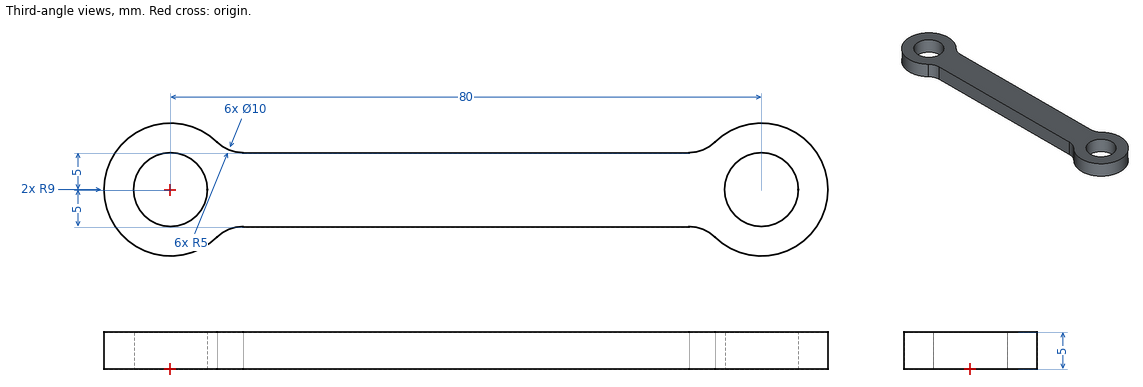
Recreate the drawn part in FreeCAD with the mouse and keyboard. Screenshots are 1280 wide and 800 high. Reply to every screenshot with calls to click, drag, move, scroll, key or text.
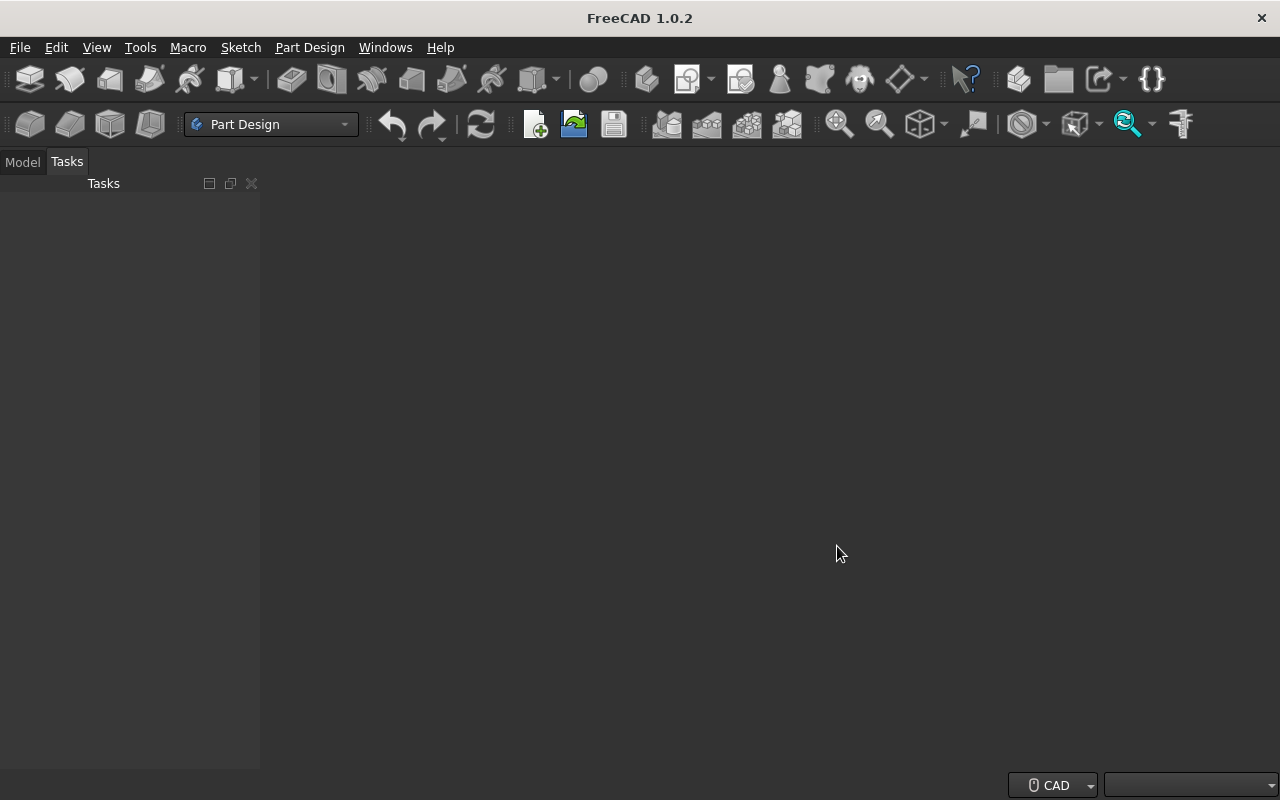
key(ctrl+n)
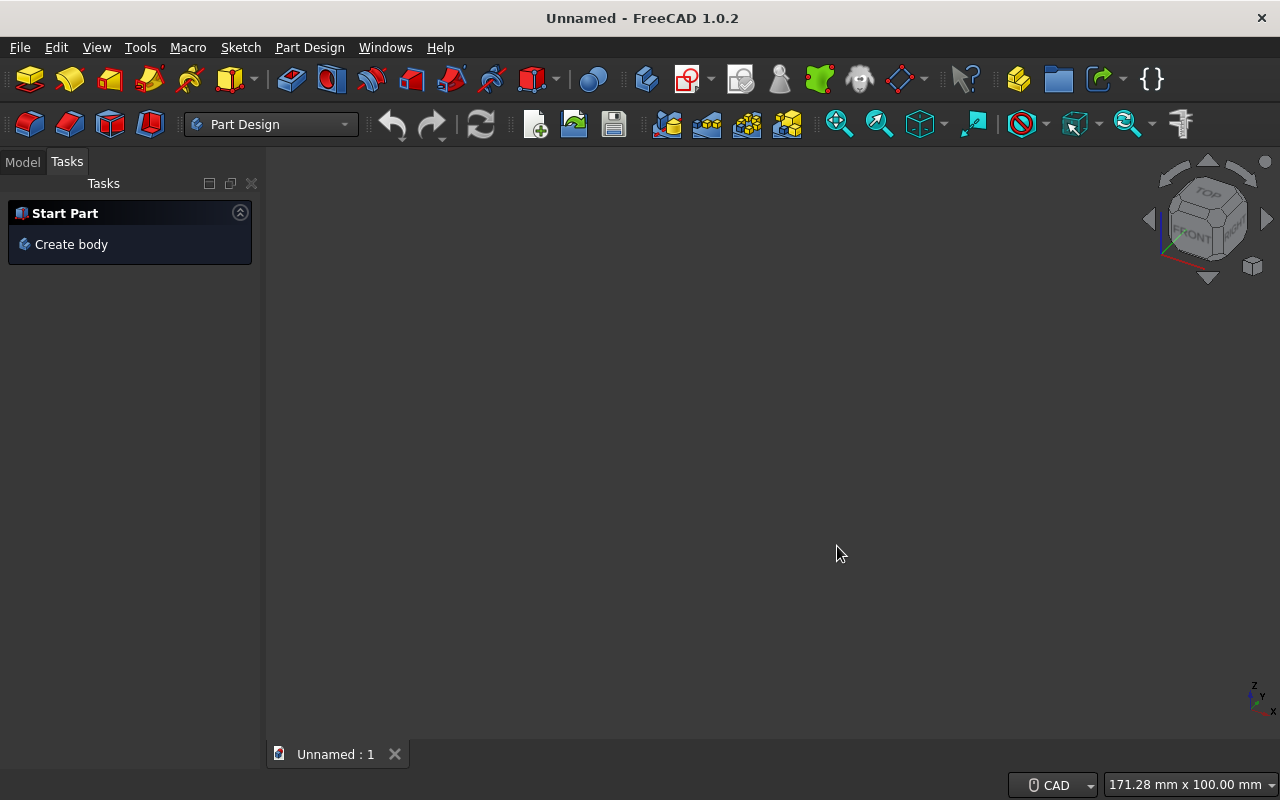
click(688, 80)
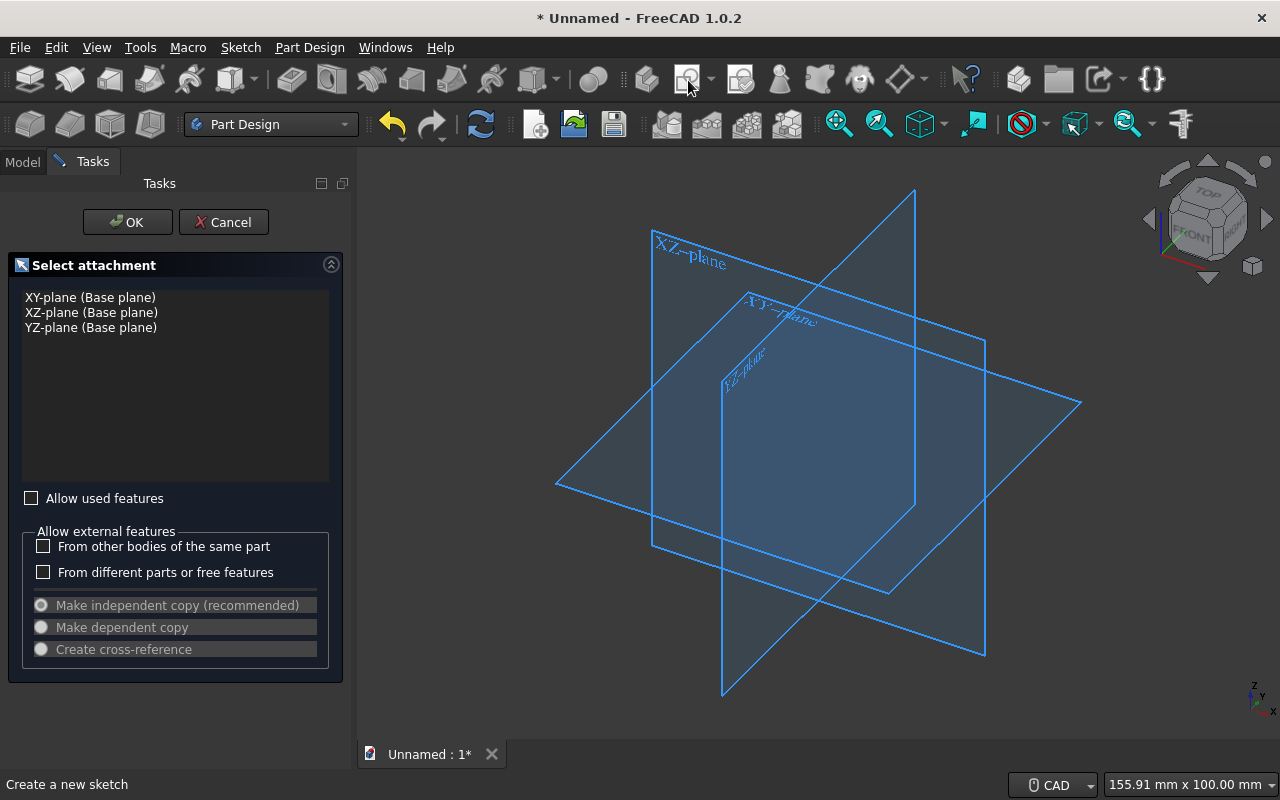
click(82, 298)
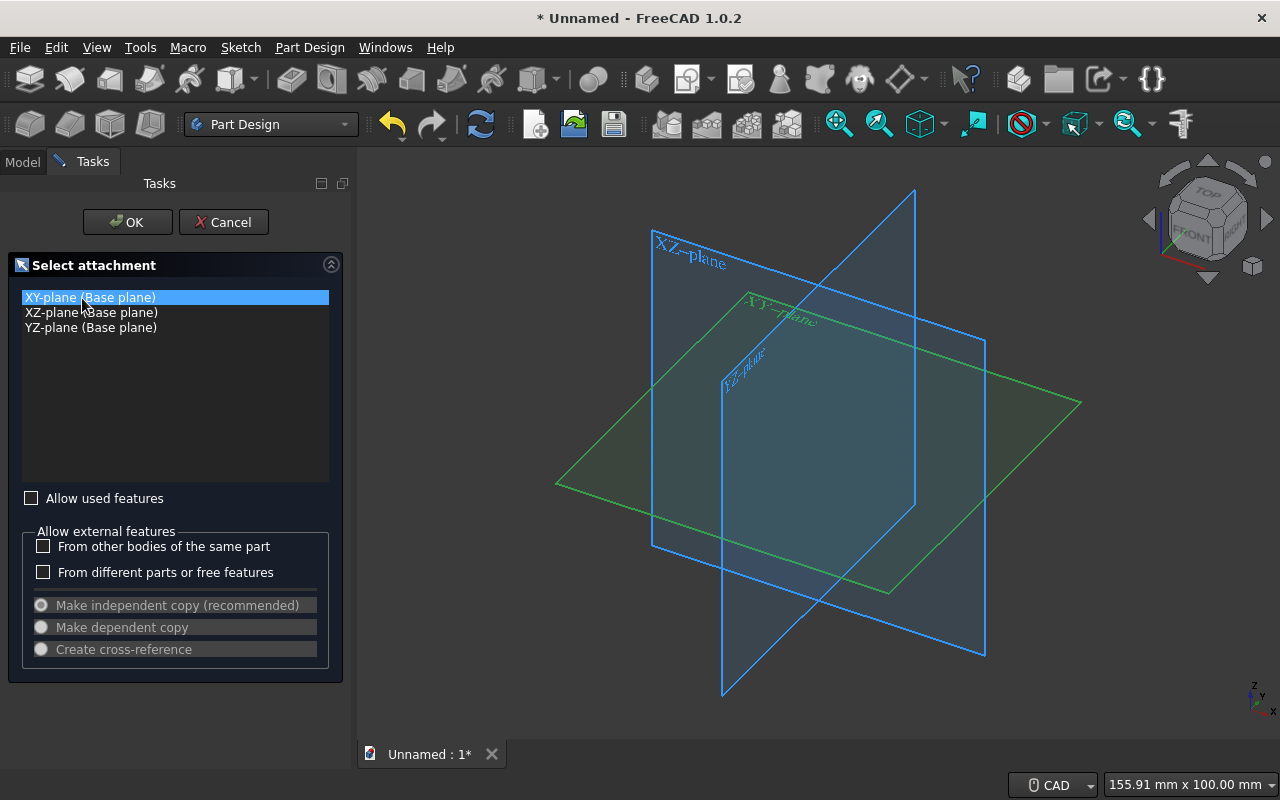
click(128, 222)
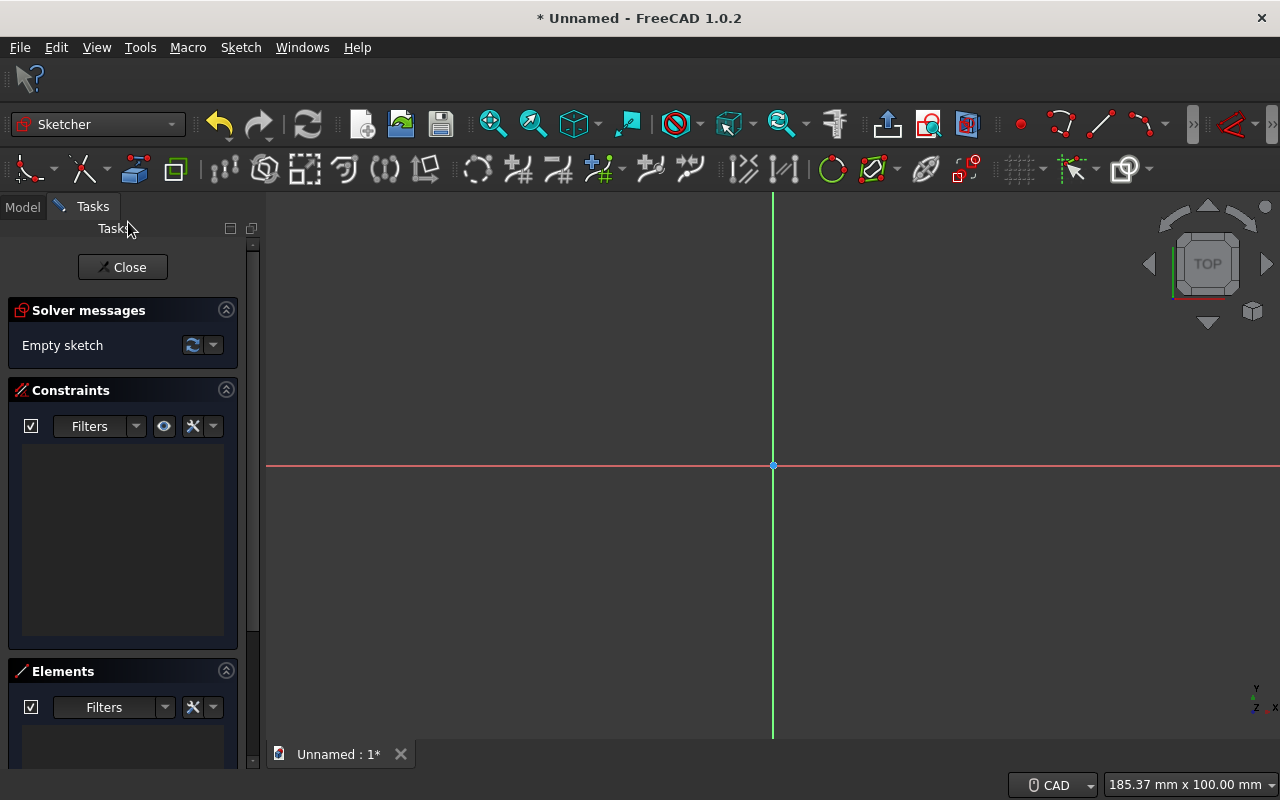
scroll(294, 465, down, 1)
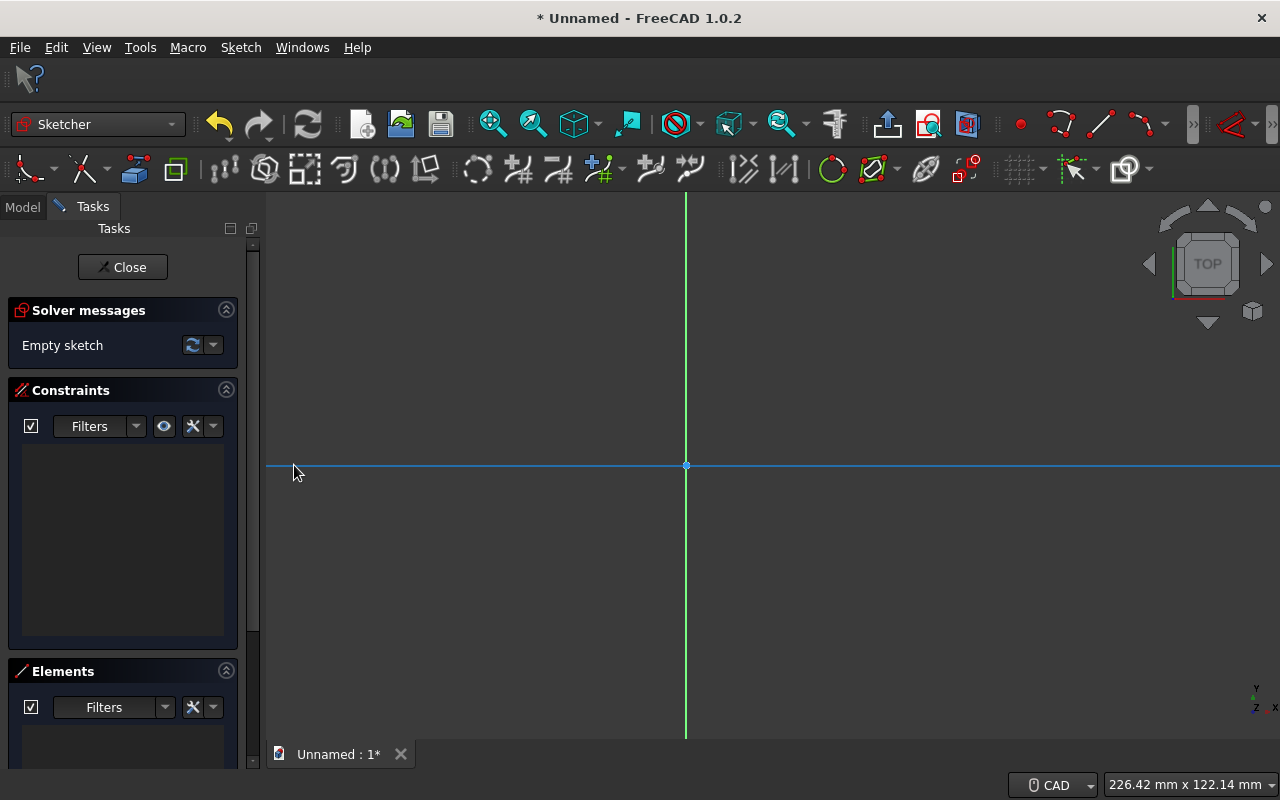
key(g)
key(l)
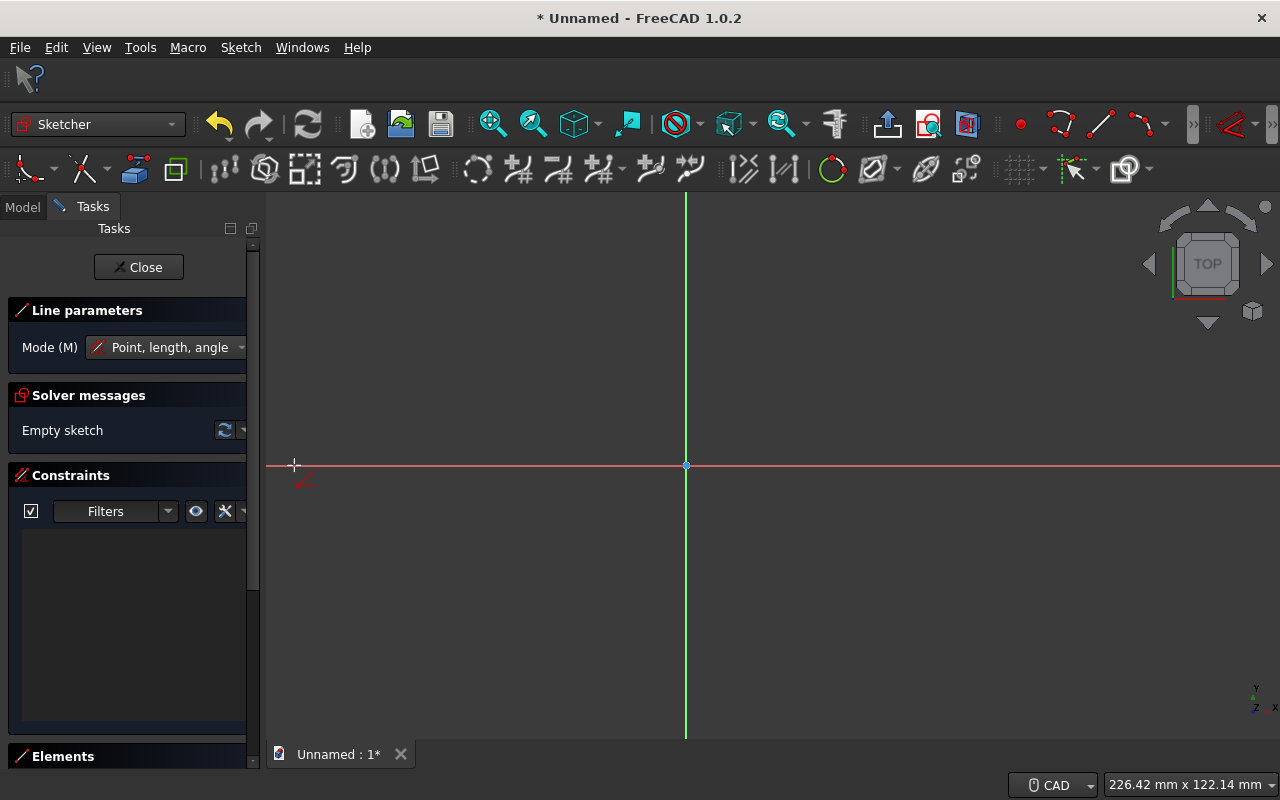
click(1001, 443)
click(730, 443)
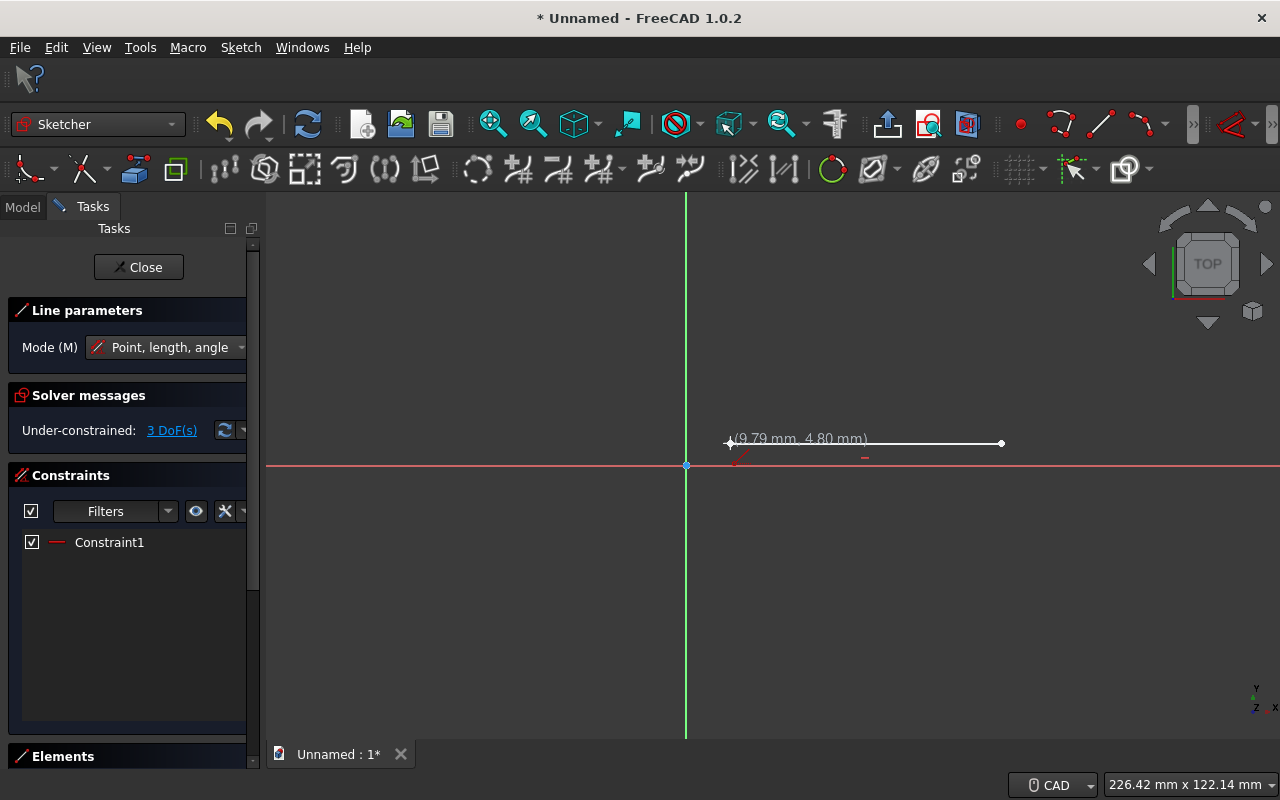
click(730, 488)
click(1001, 488)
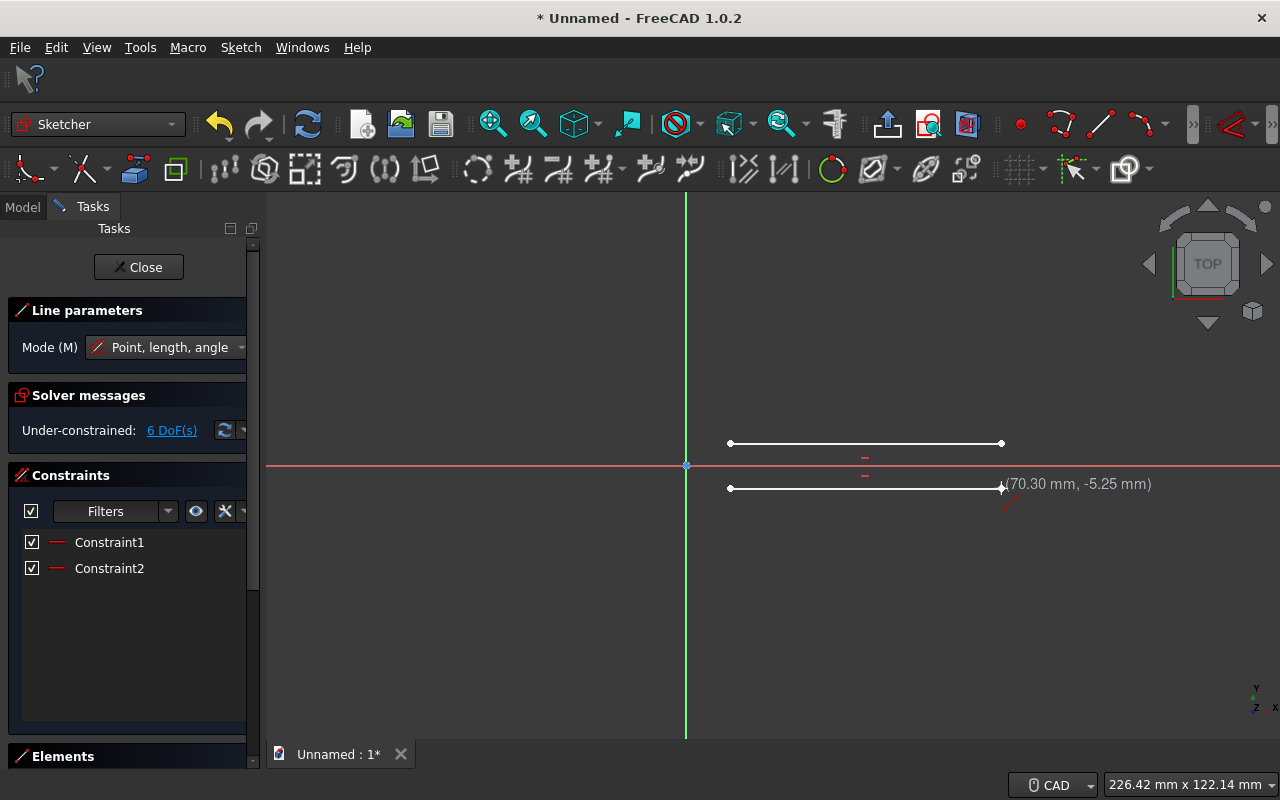
key(g)
key(3)
key(a)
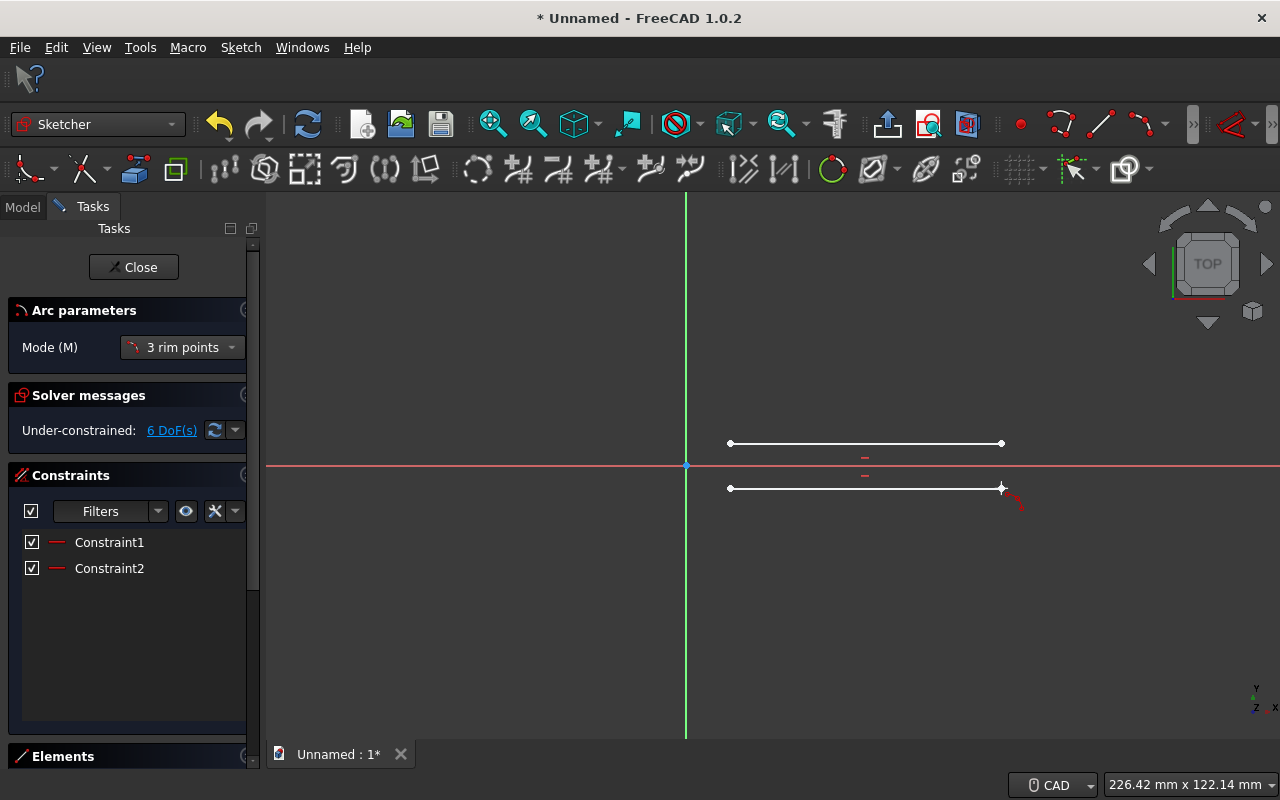
click(730, 444)
click(714, 437)